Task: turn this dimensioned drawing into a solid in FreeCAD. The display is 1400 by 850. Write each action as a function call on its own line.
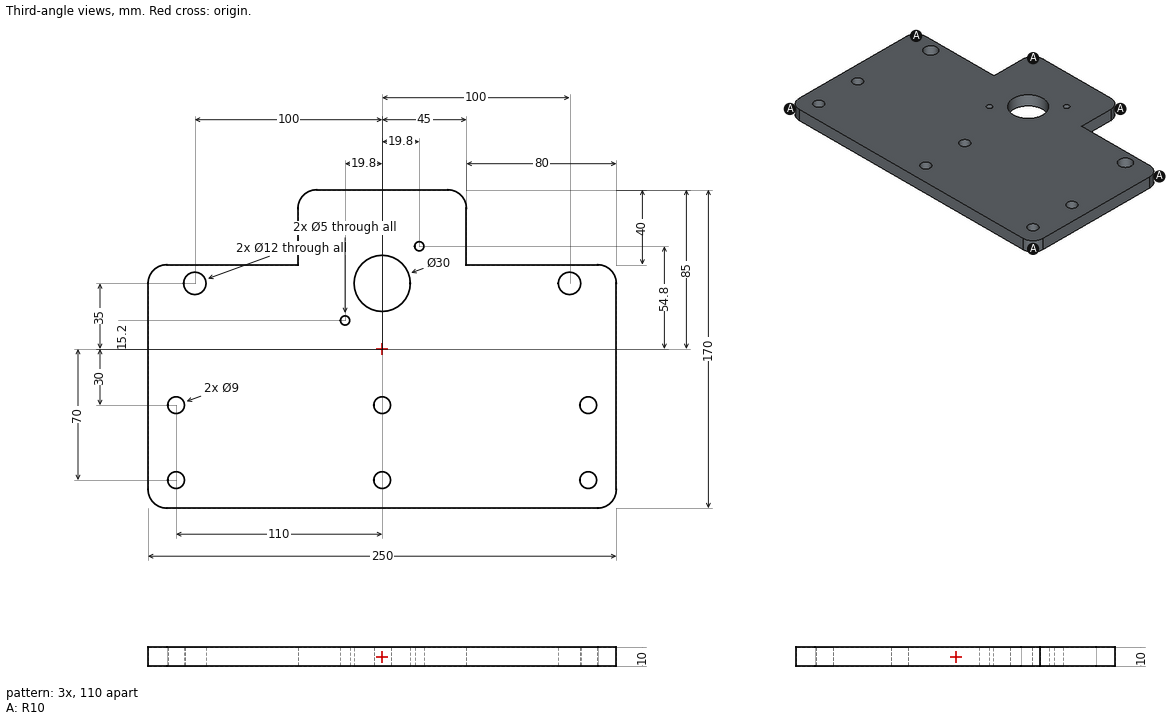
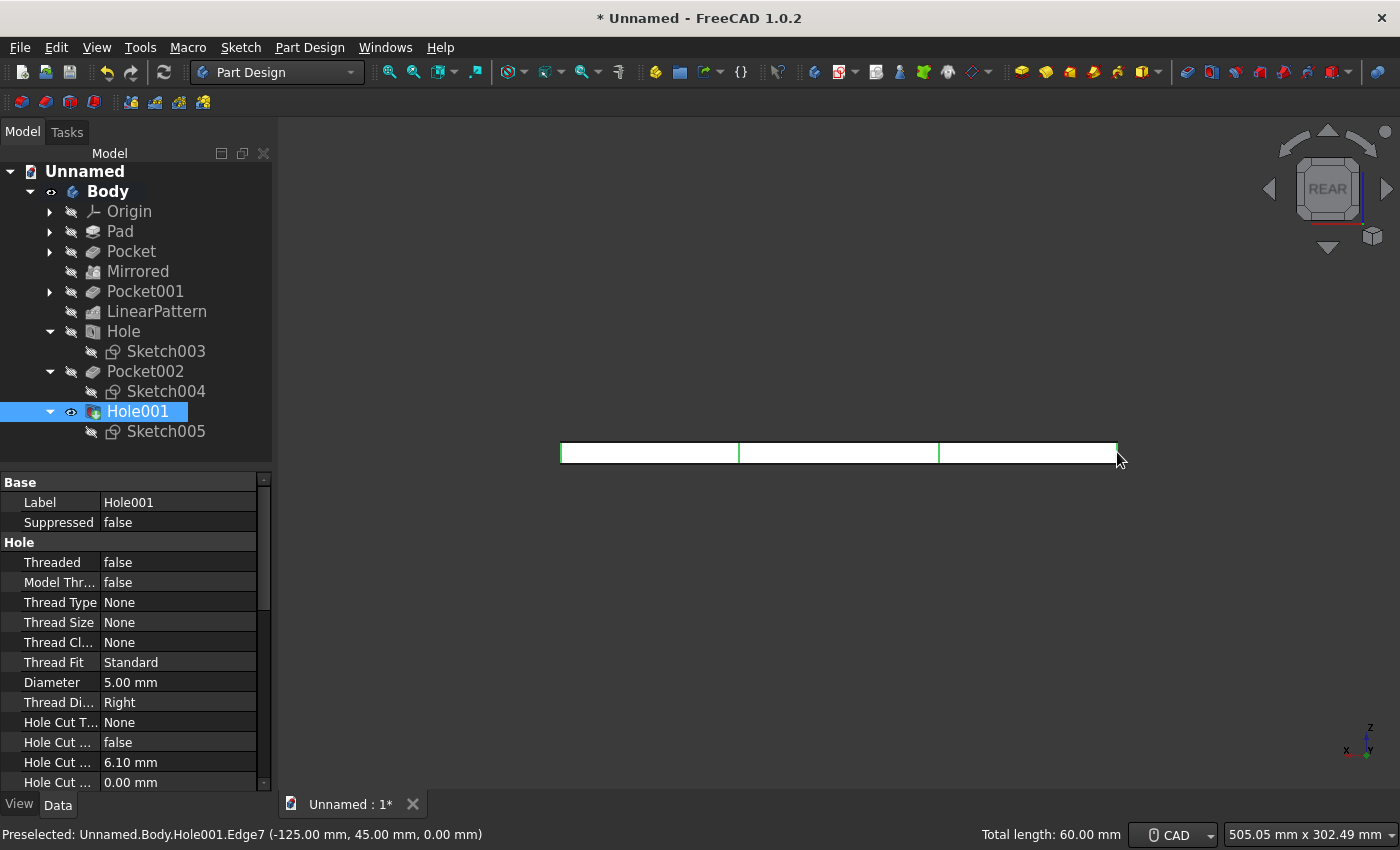
click(22, 102)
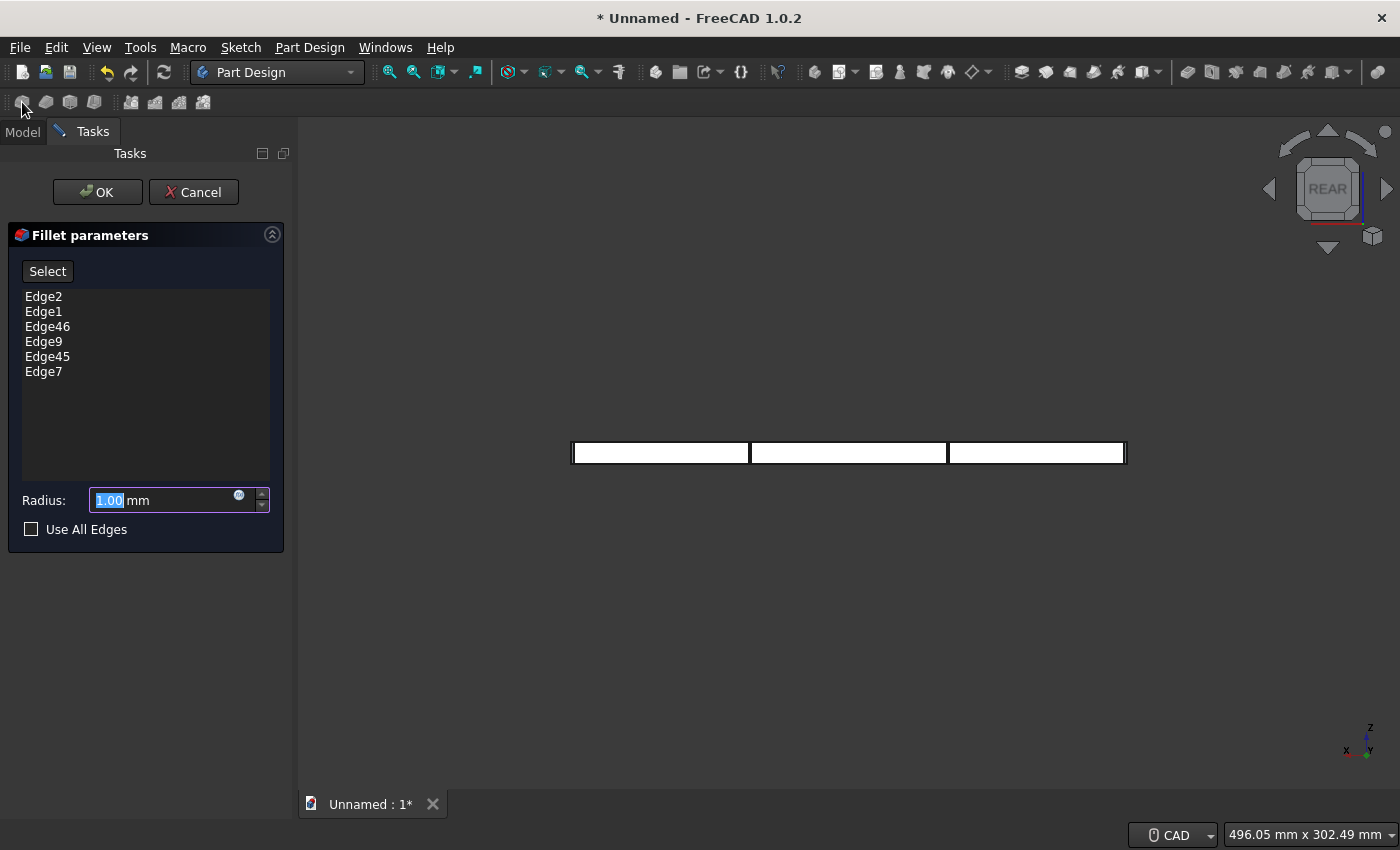
text(10)
key(Tab)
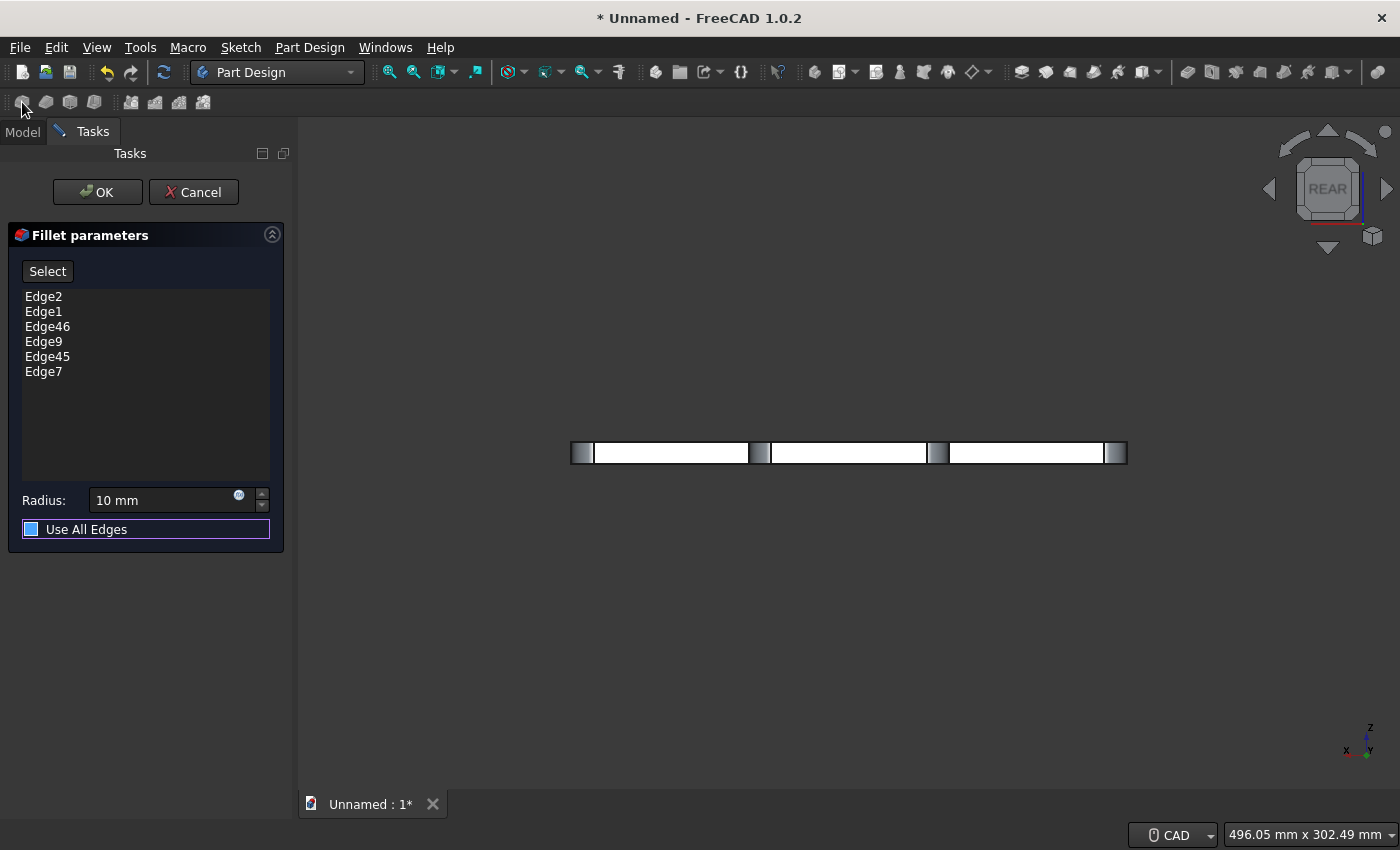
click(98, 192)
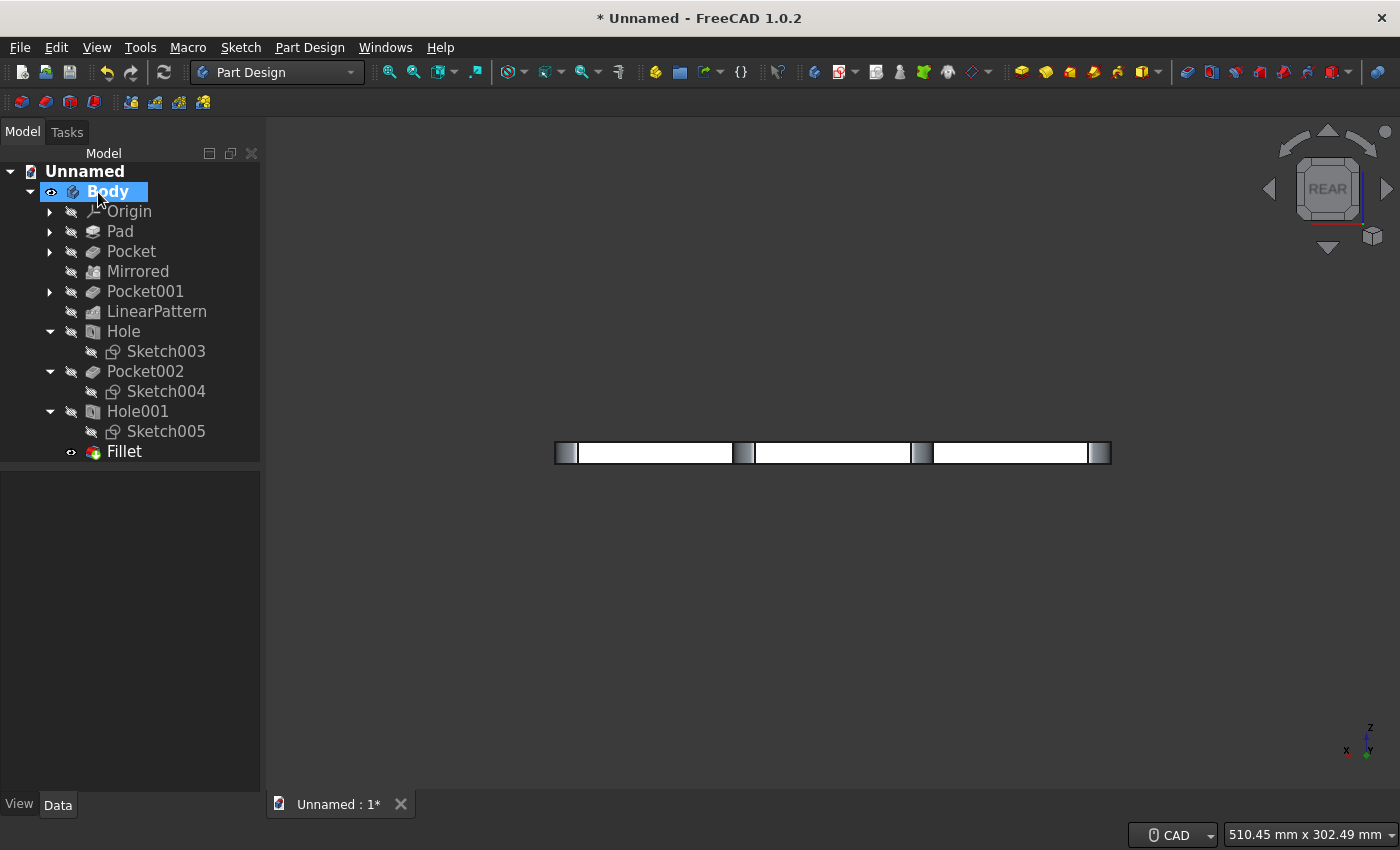
key(0)